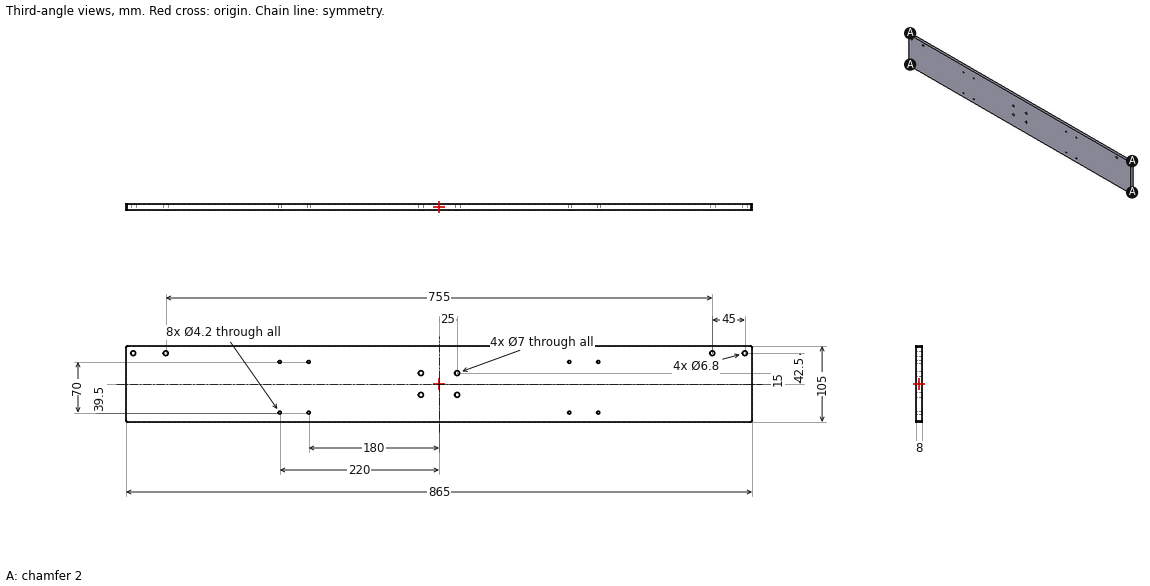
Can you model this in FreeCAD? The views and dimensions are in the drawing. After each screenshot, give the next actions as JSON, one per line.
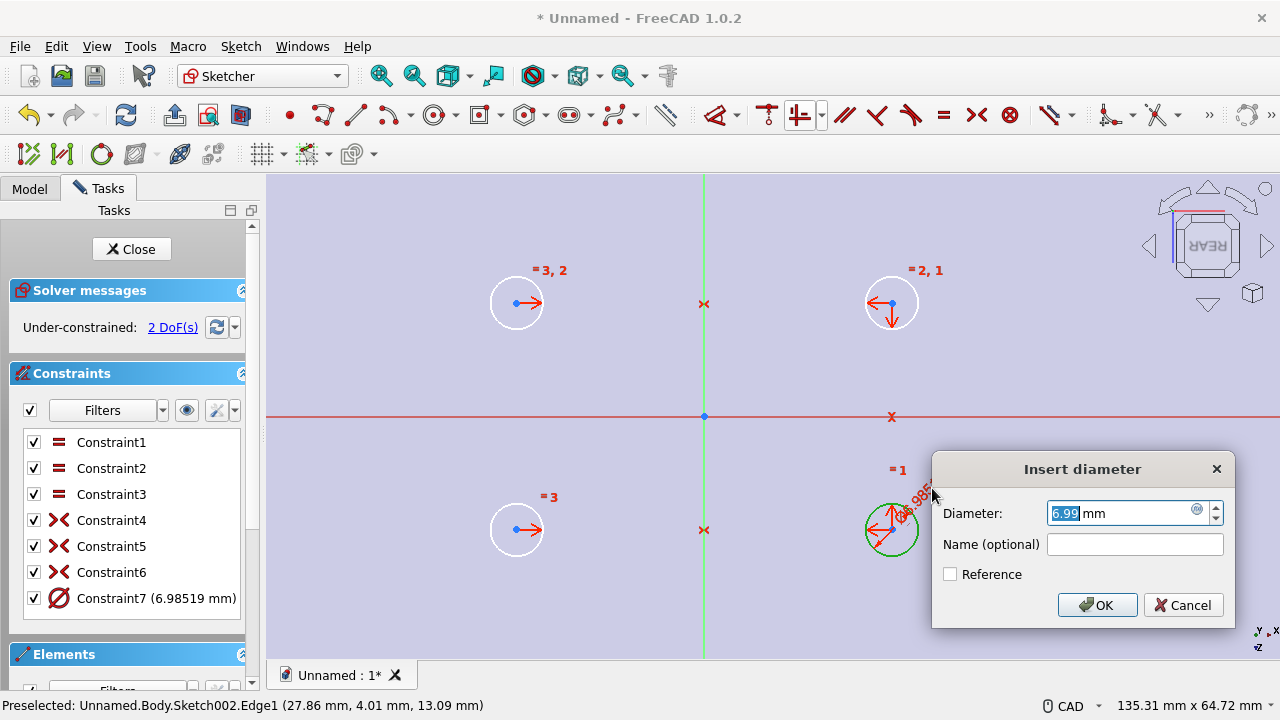
{"action": "type", "text": "7"}
{"action": "key", "text": "Return"}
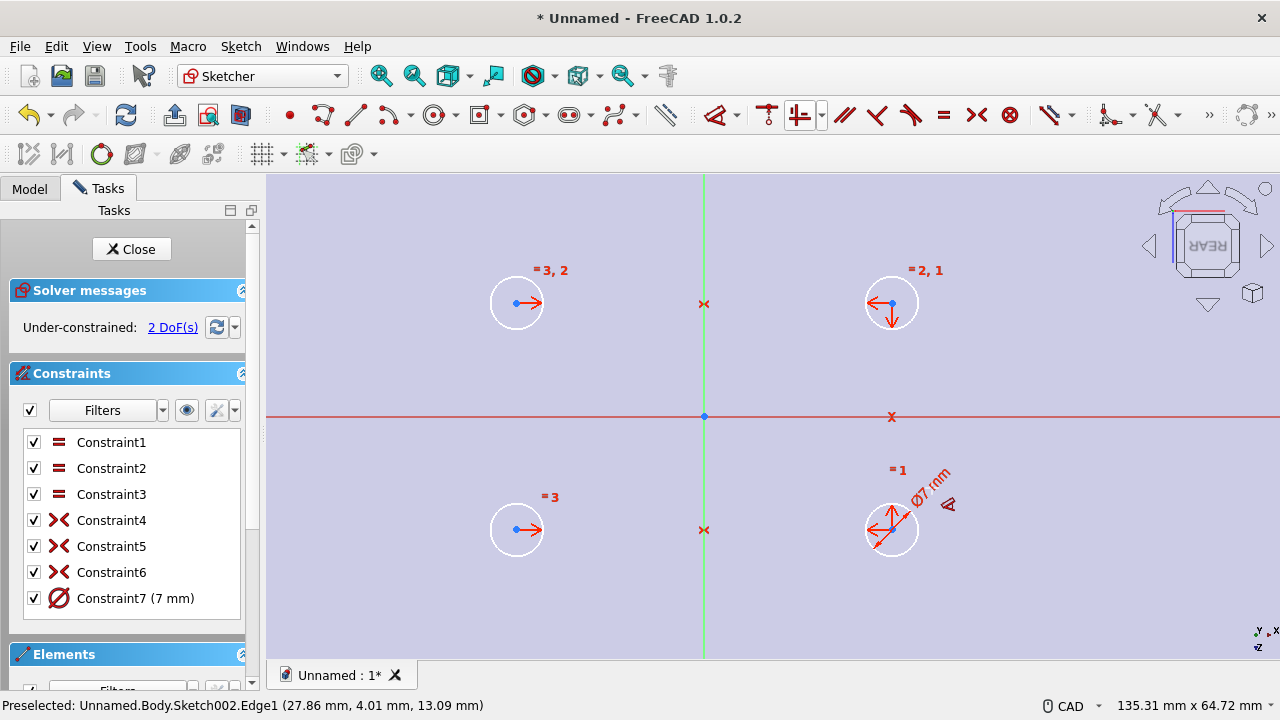
{"action": "left_click", "coordinate": [892, 530]}
{"action": "left_click", "coordinate": [798, 564]}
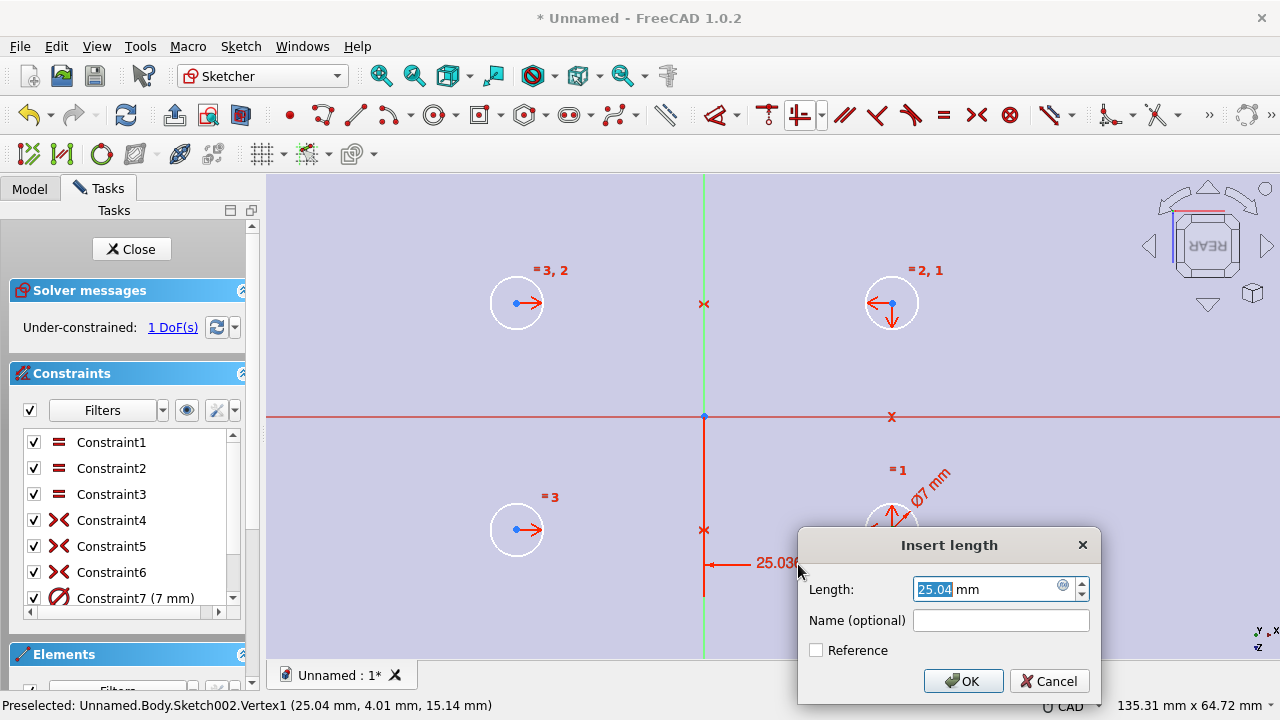
{"action": "type", "text": "25"}
{"action": "key", "text": "Return"}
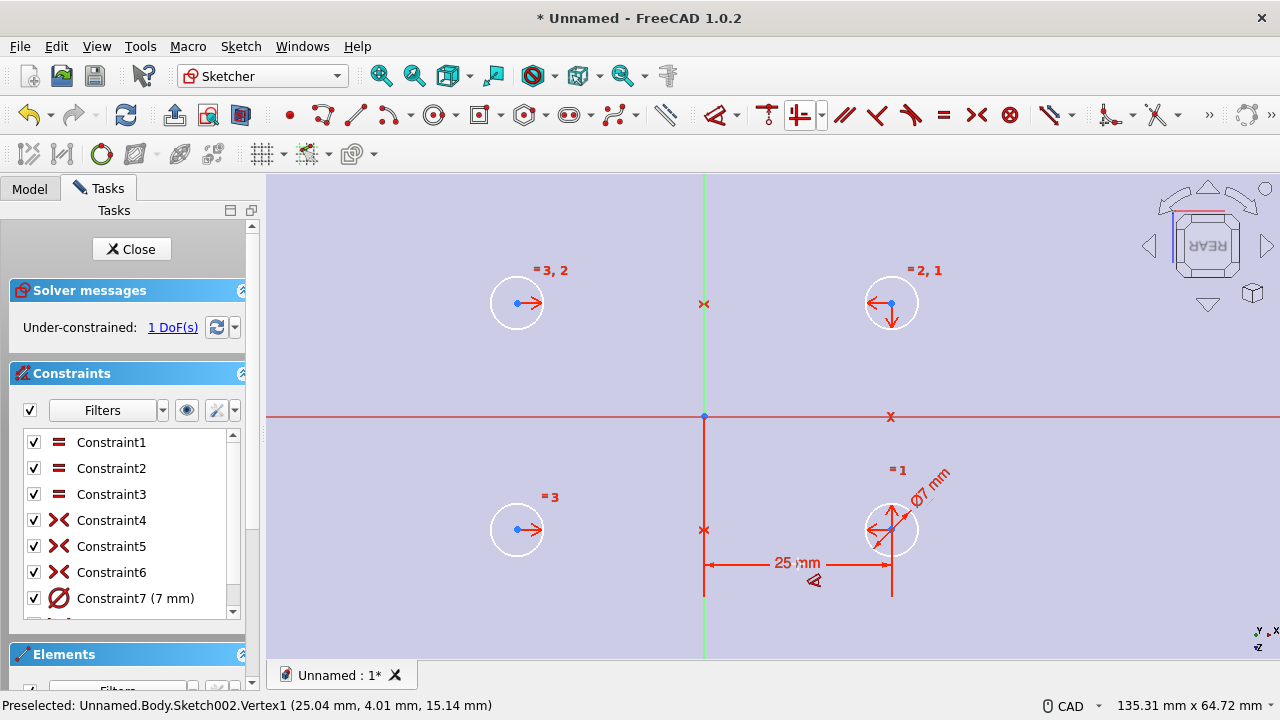
{"action": "left_click", "coordinate": [892, 530]}
{"action": "left_click", "coordinate": [926, 447]}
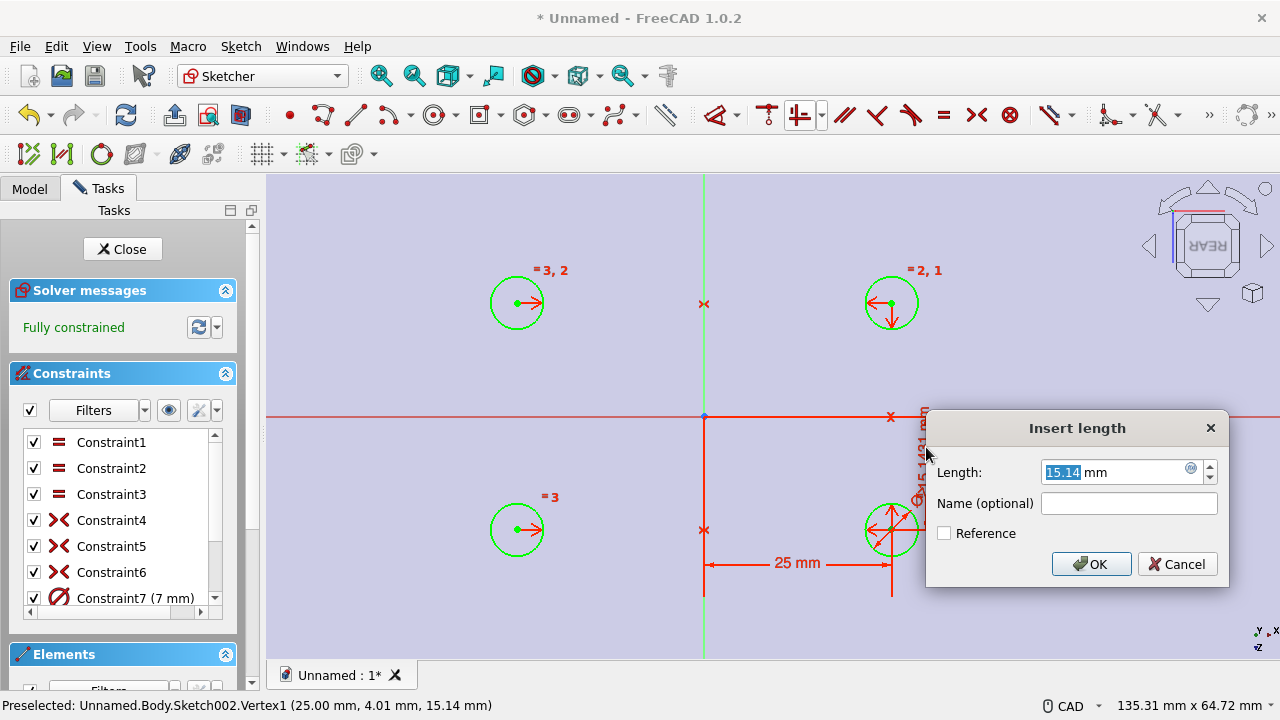
{"action": "type", "text": "15"}
{"action": "key", "text": "Return"}
{"action": "key", "text": "Escape"}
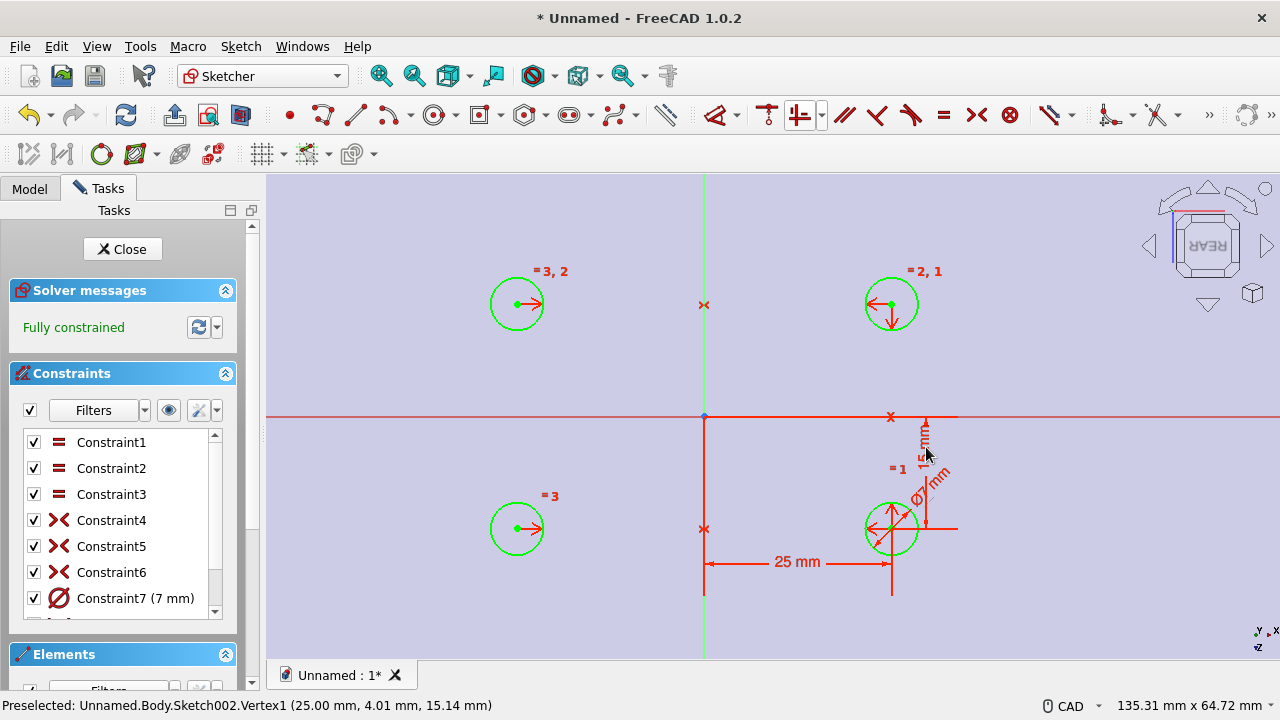
{"action": "left_click", "coordinate": [123, 249]}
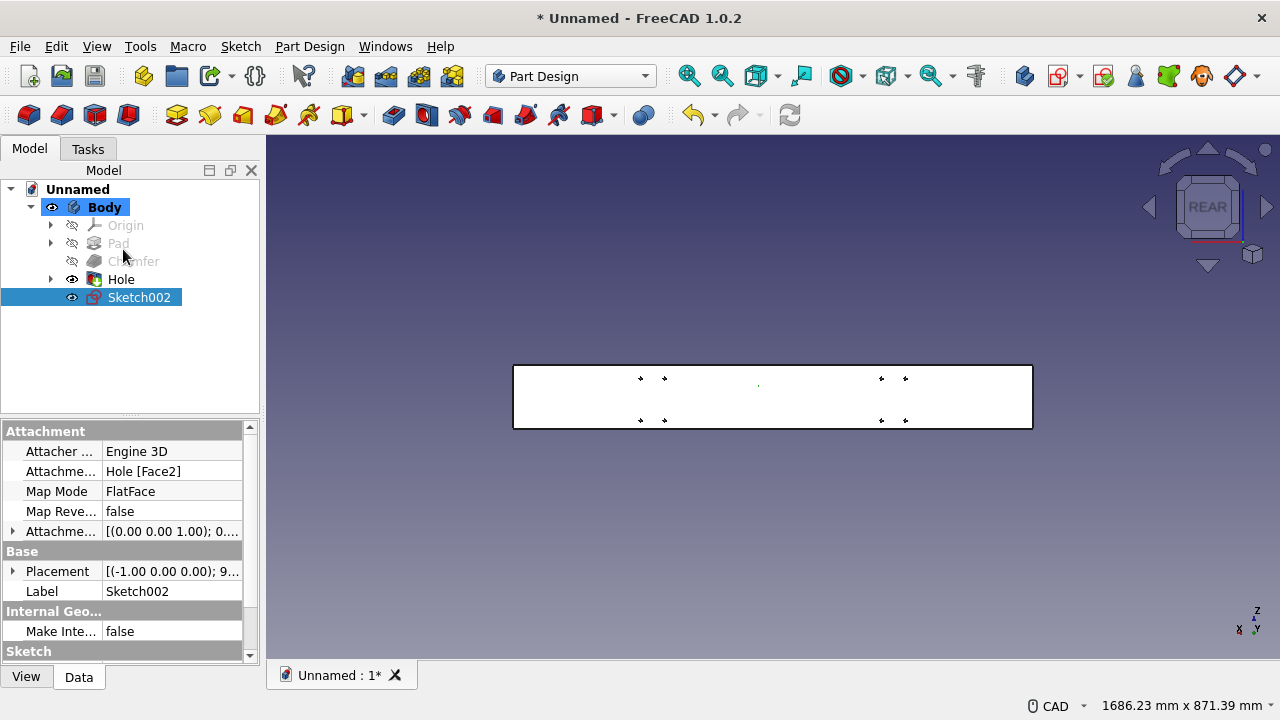
{"action": "left_click", "coordinate": [427, 116]}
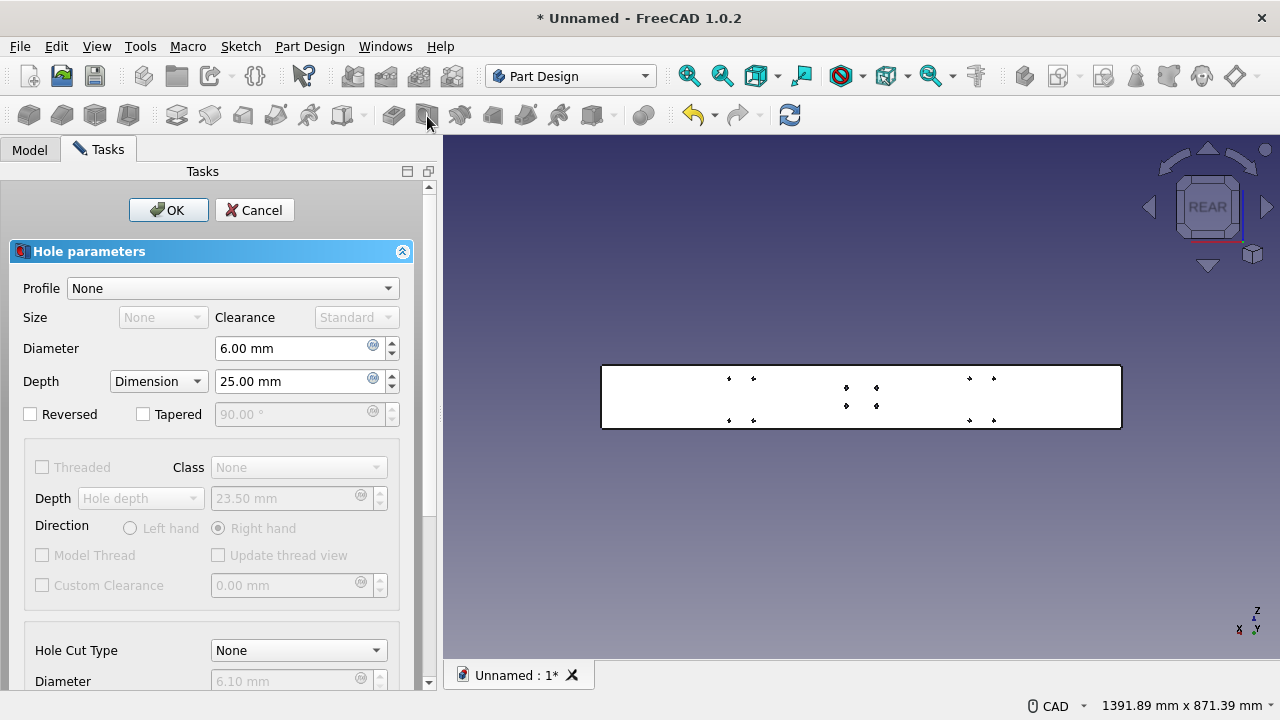
{"action": "triple_click", "coordinate": [300, 348]}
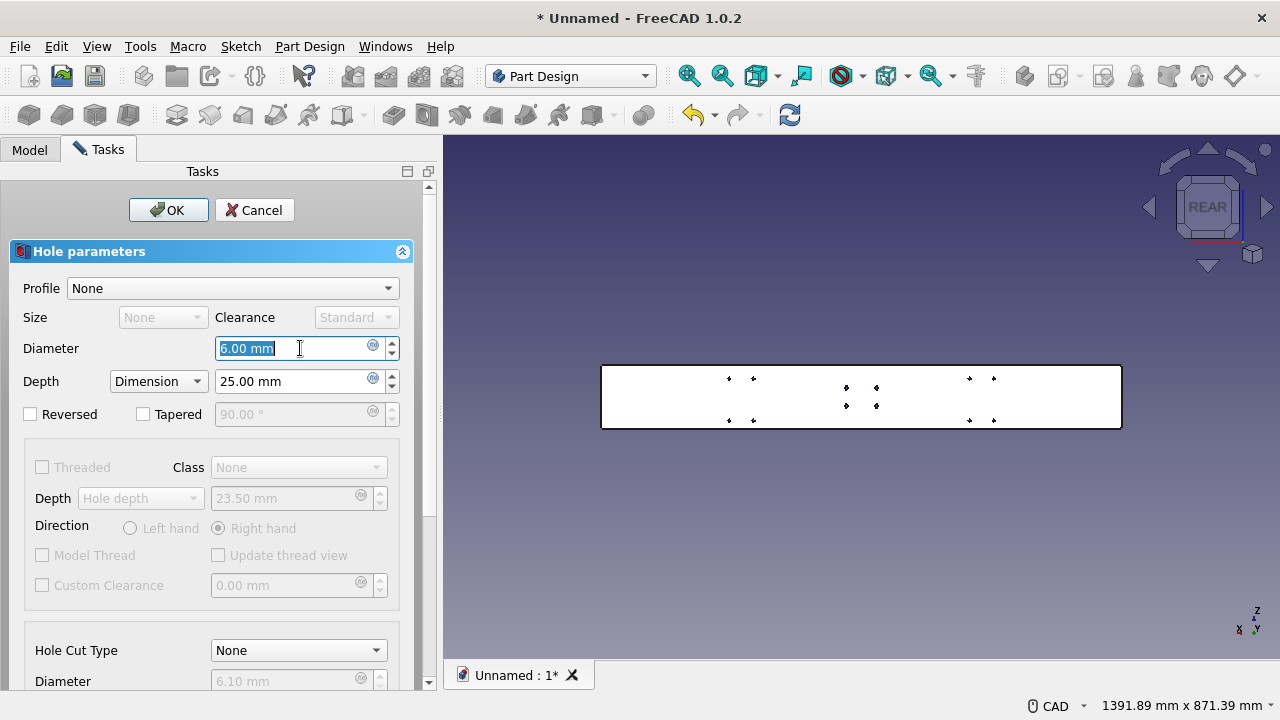
{"action": "type", "text": "7"}
{"action": "key", "text": "Tab"}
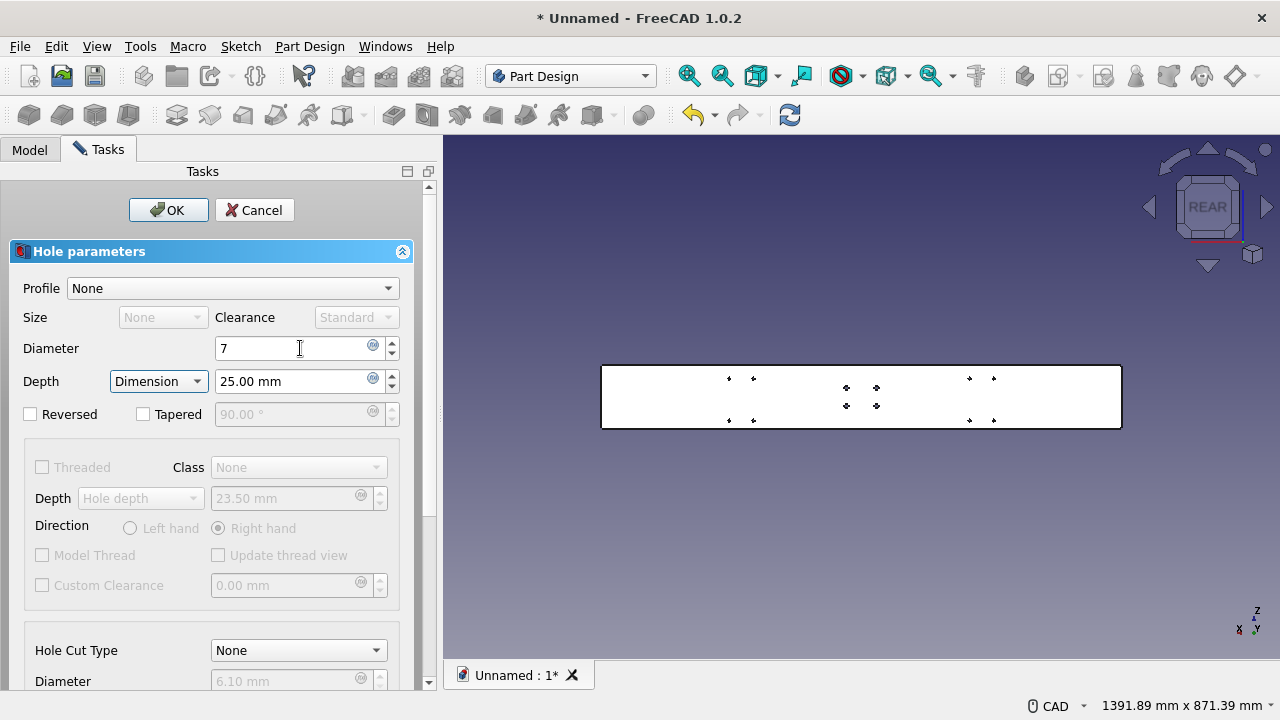
{"action": "left_click", "coordinate": [160, 382]}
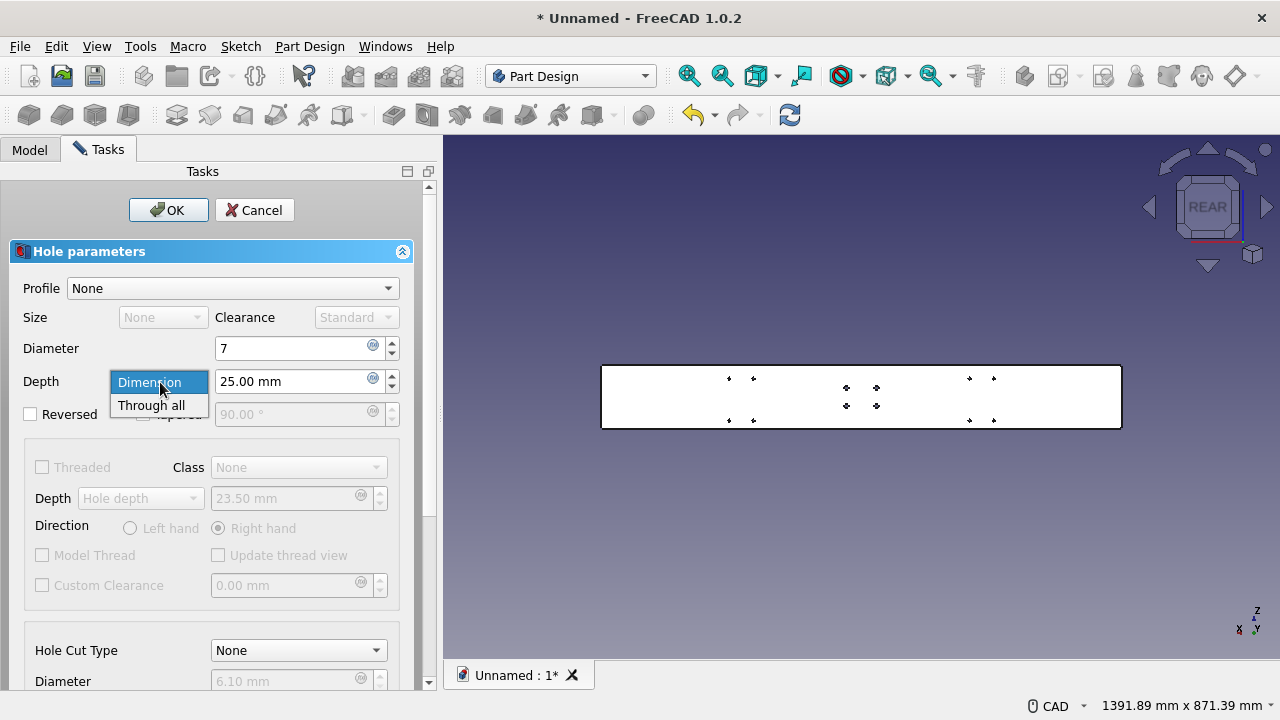
{"action": "left_click", "coordinate": [158, 406]}